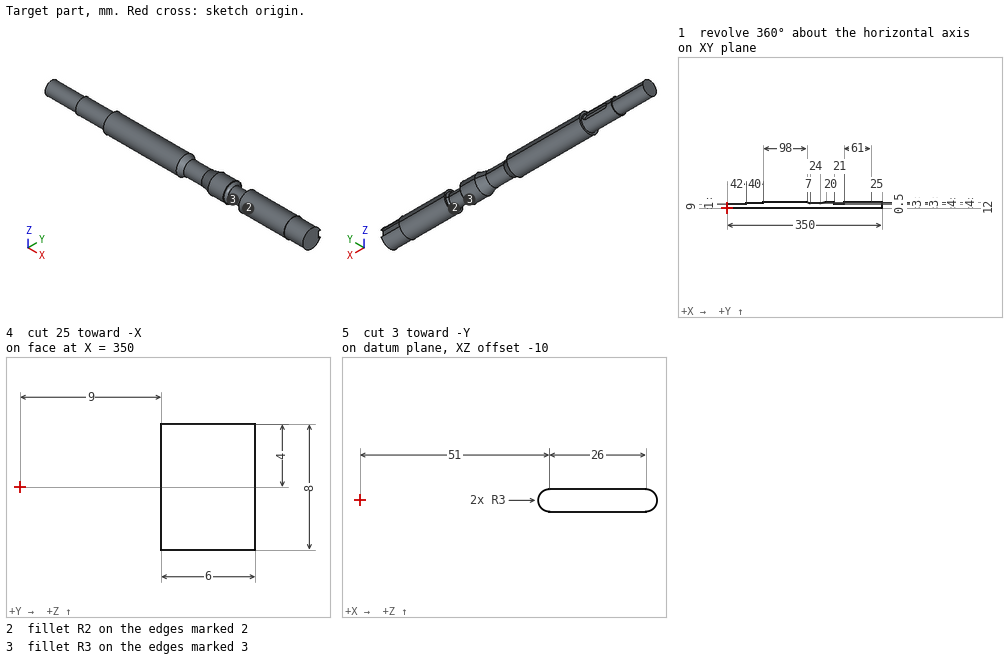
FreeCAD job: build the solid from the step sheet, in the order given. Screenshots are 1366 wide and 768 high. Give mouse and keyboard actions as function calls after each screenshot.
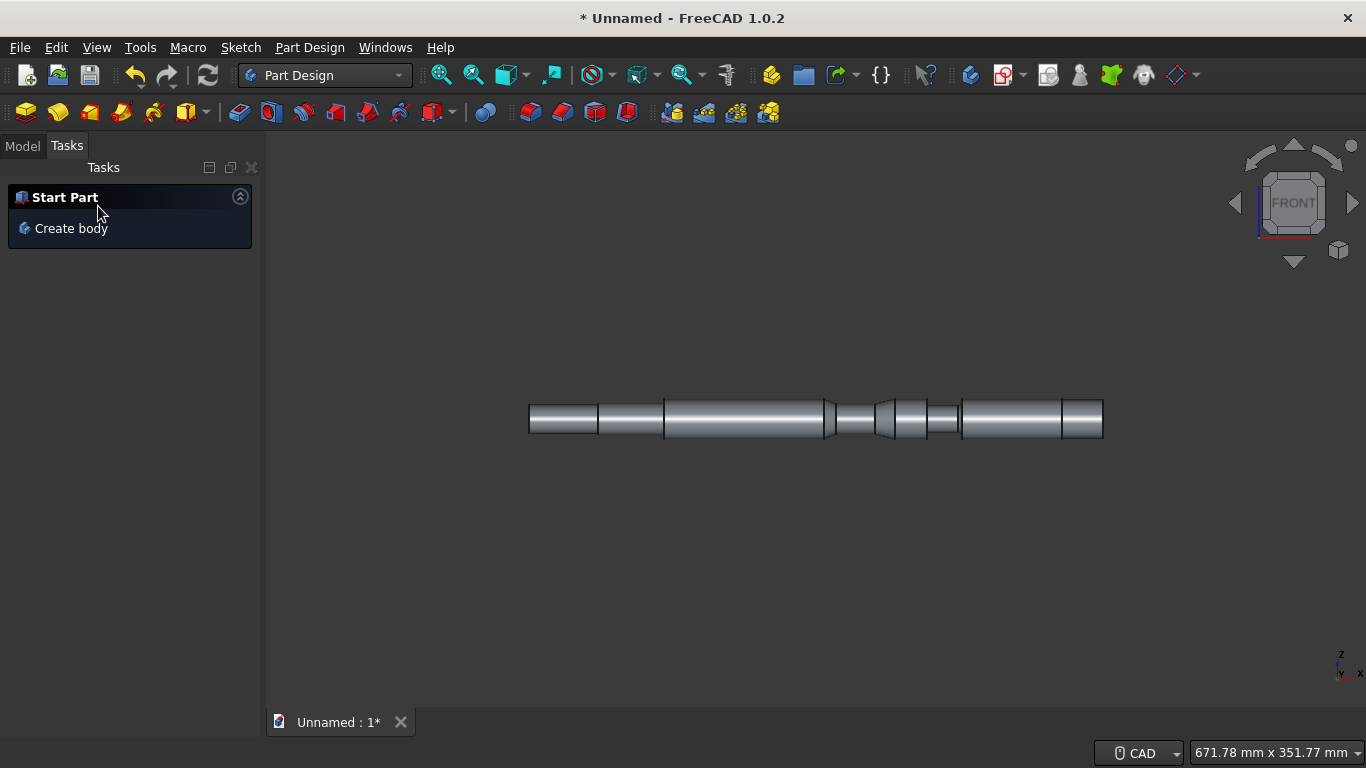
key(3)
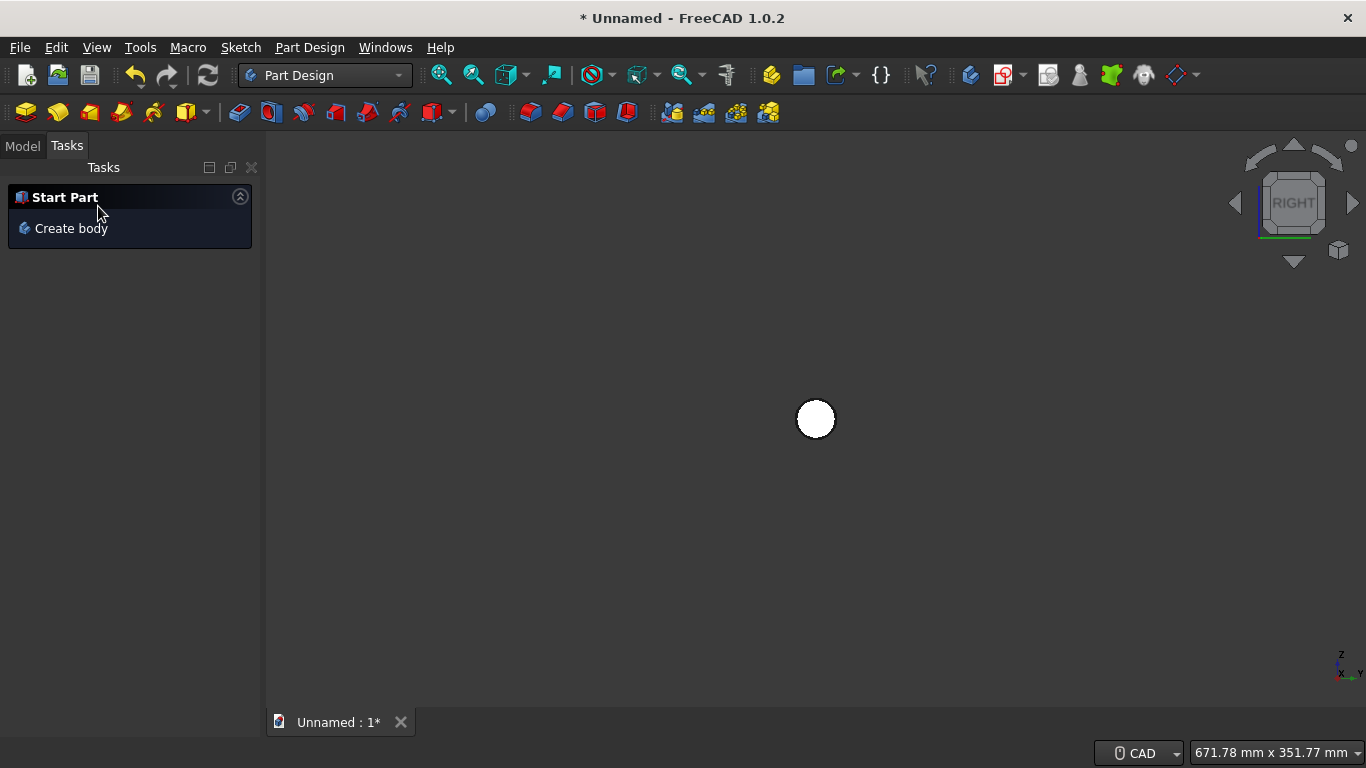
click(442, 76)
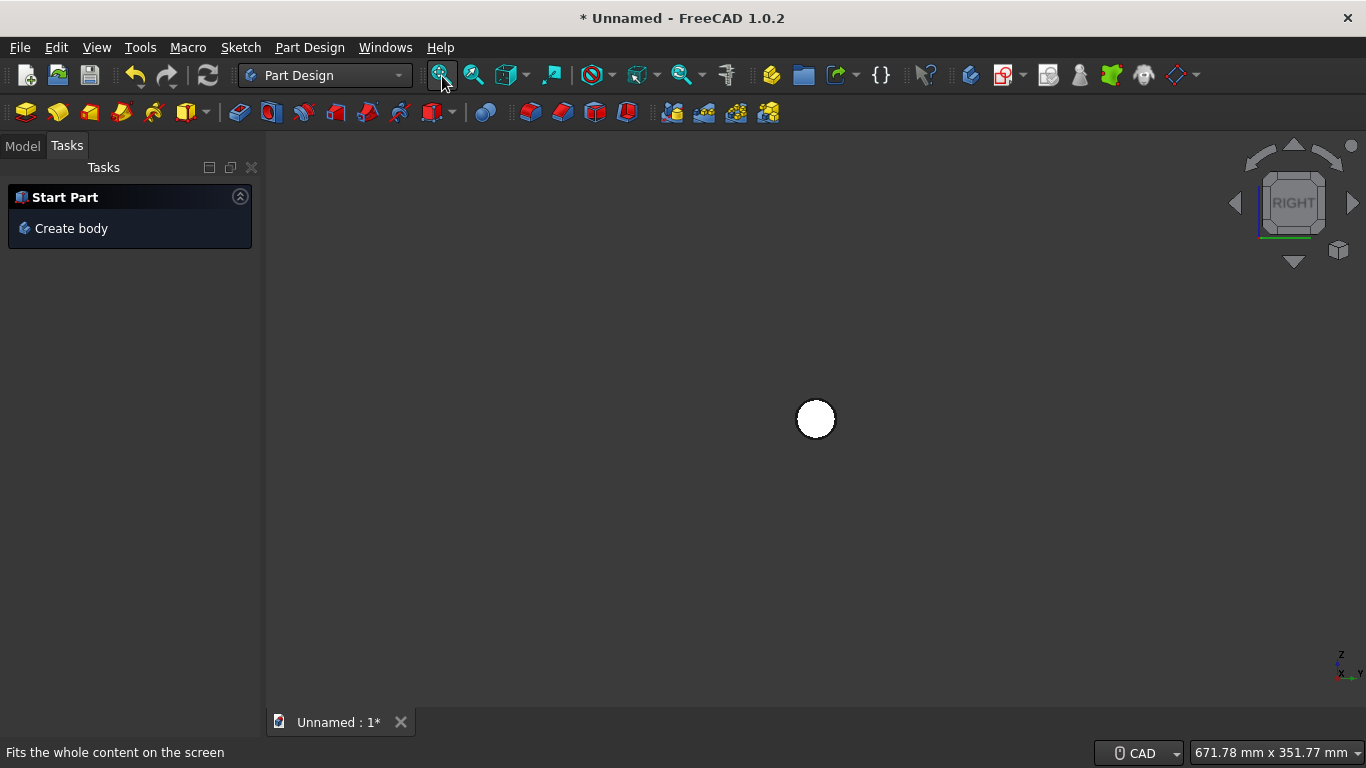
key(5)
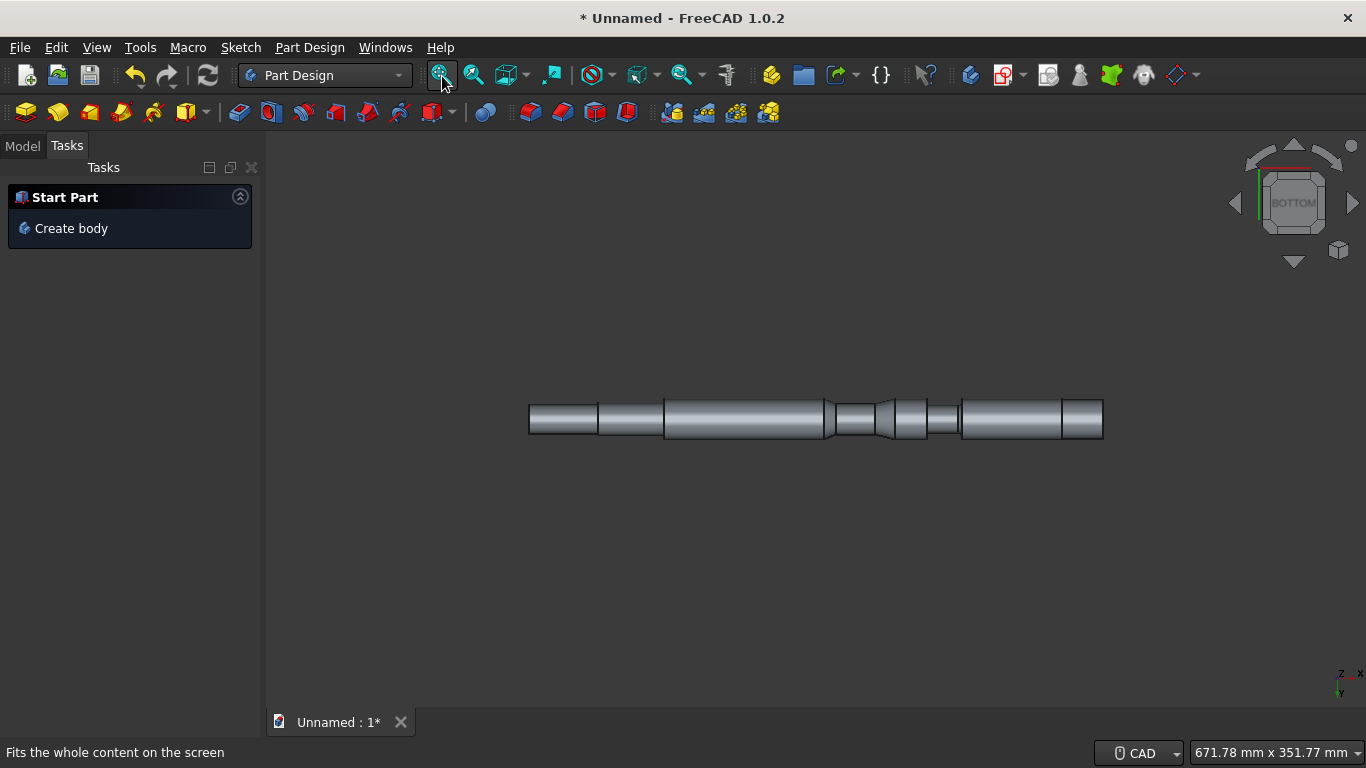
key(4)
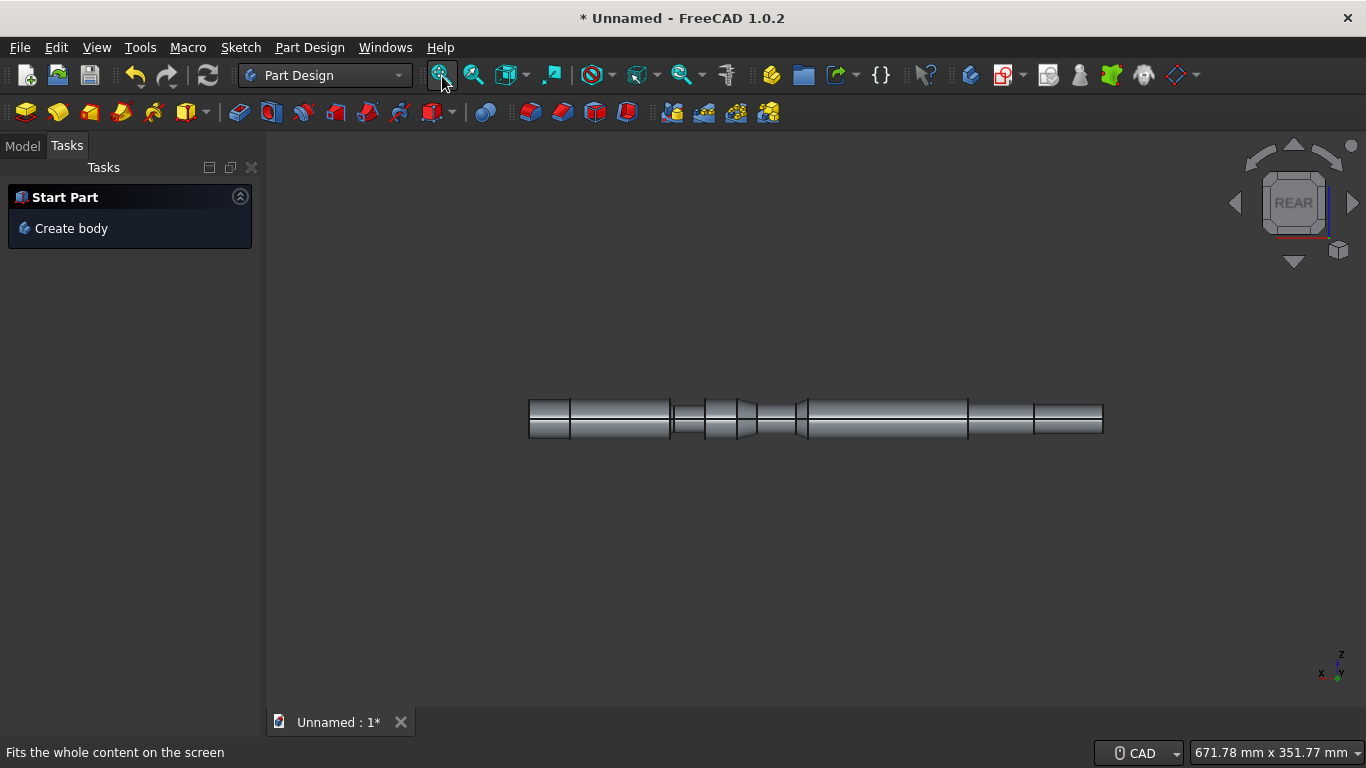
key(6)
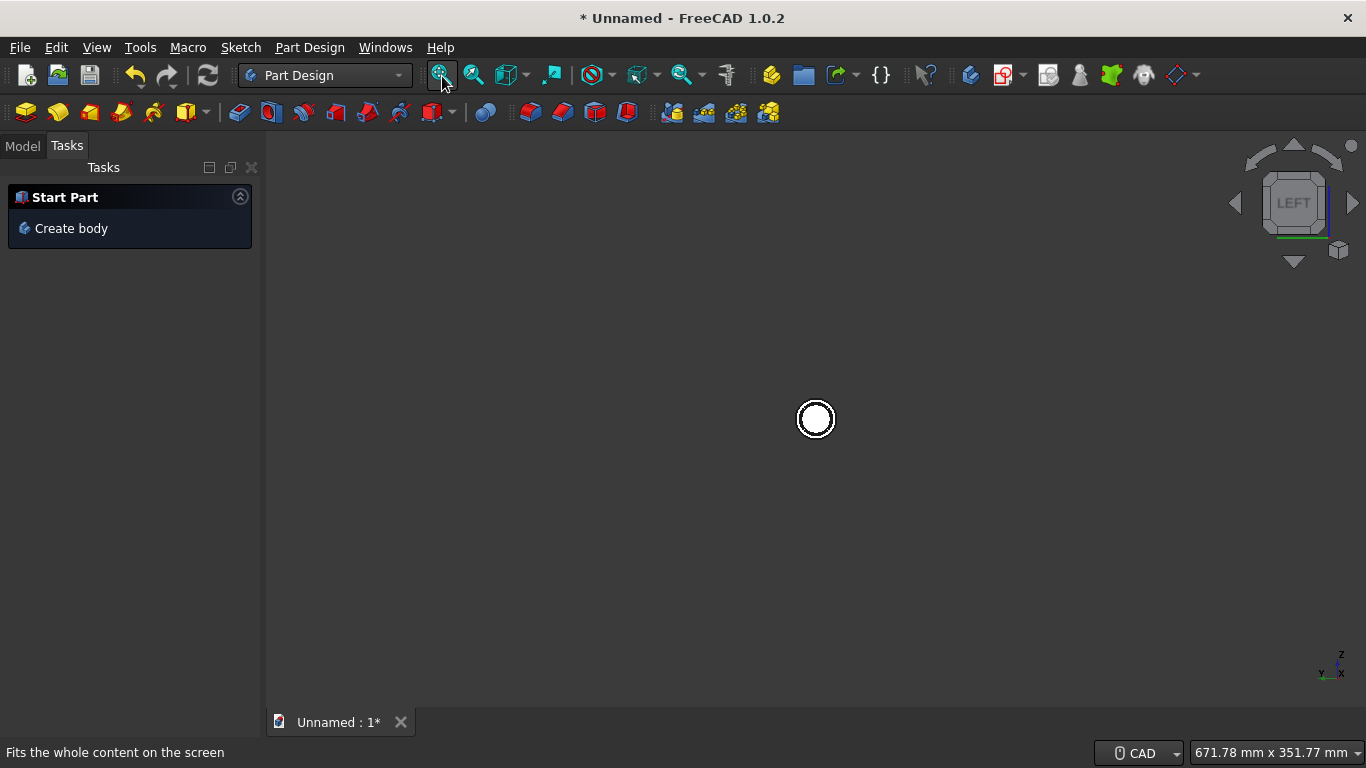
click(442, 76)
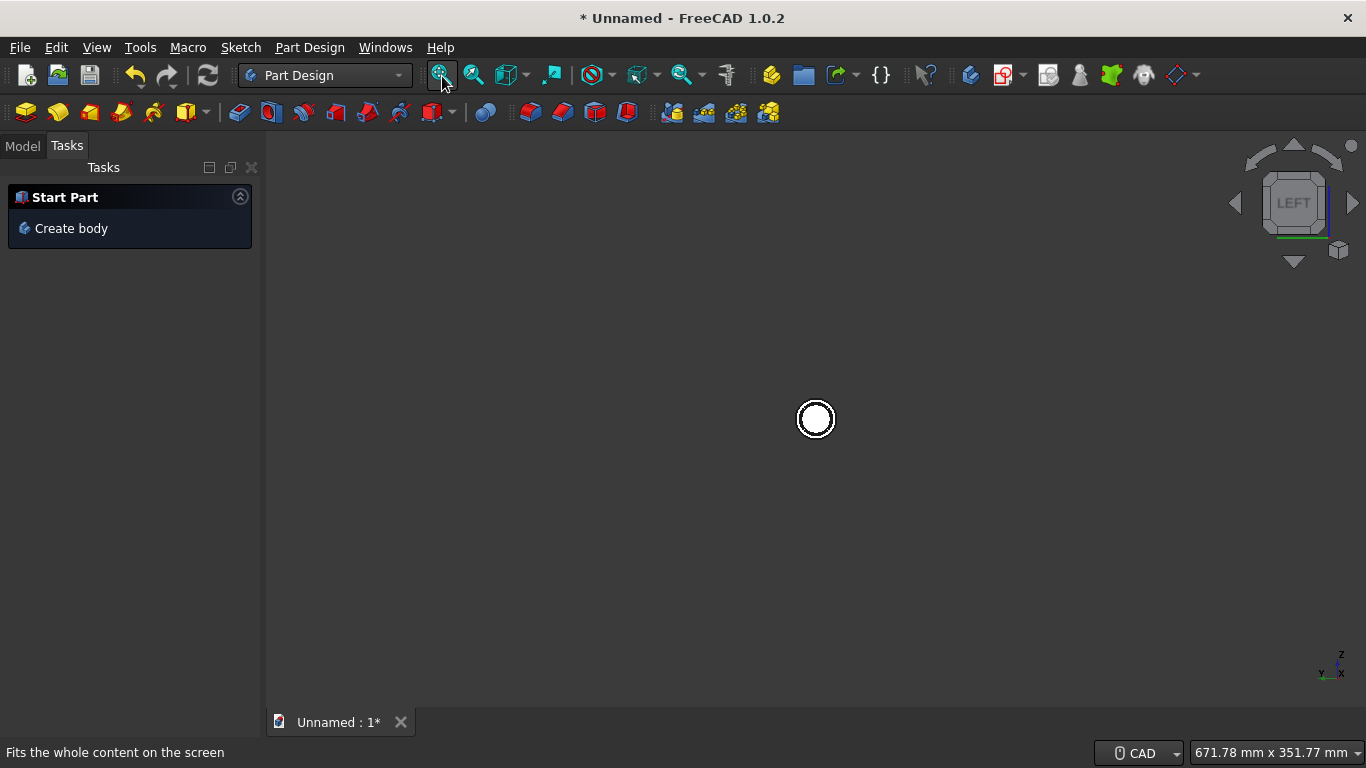
key(v)
key(3)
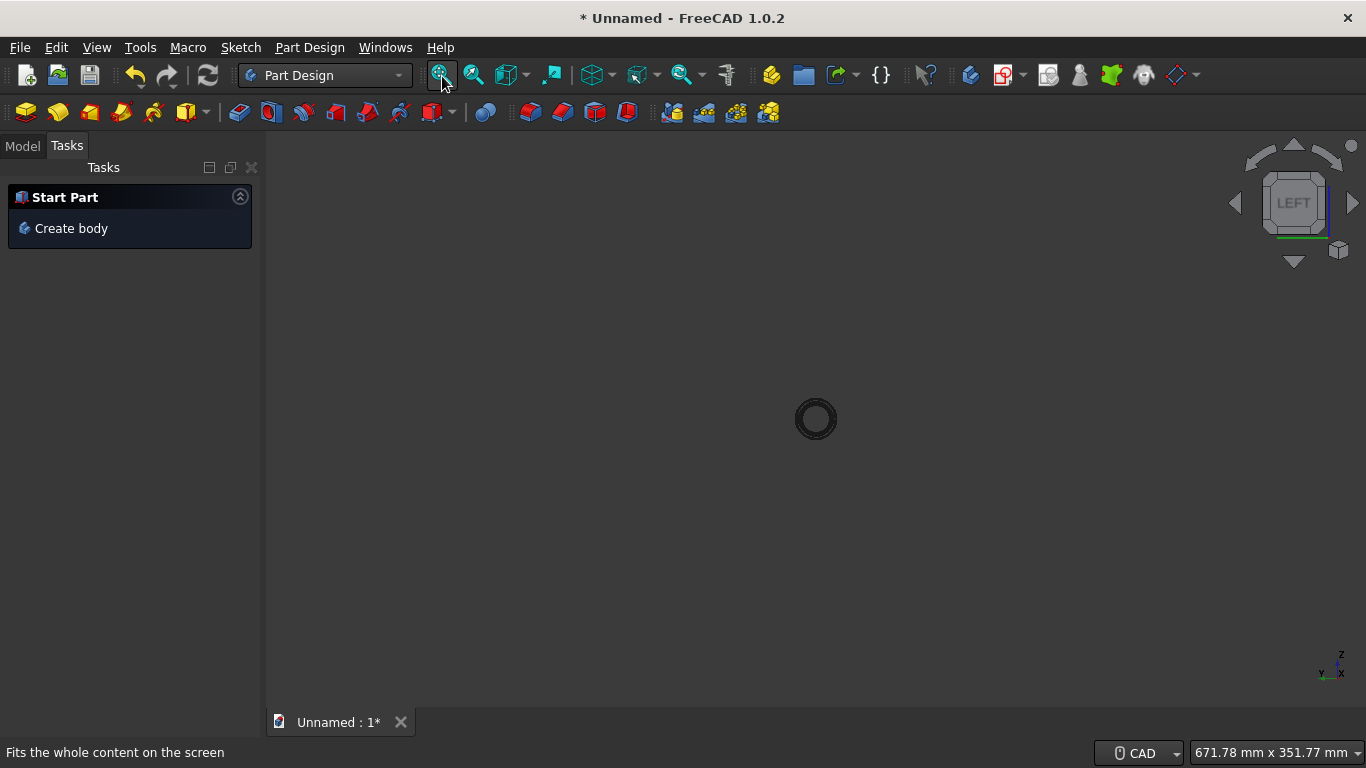
key(0)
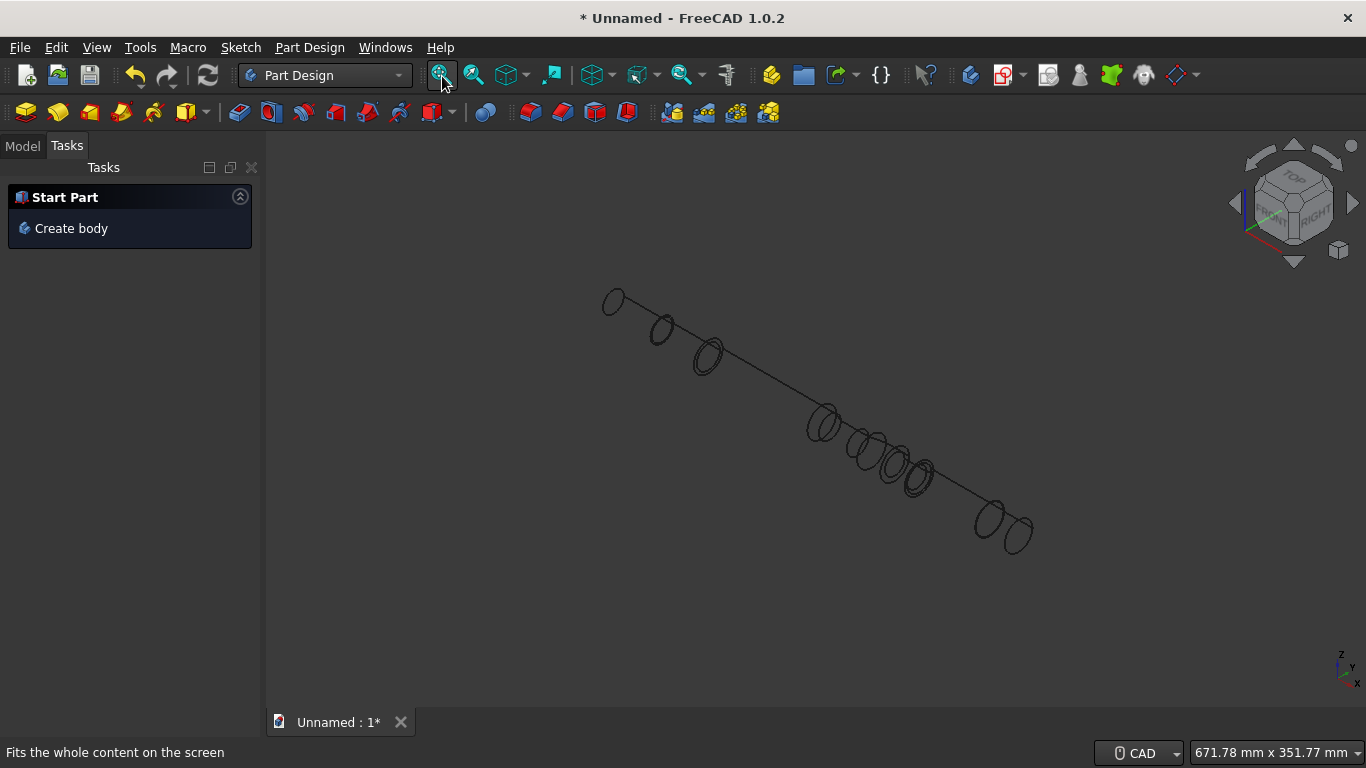
click(892, 476)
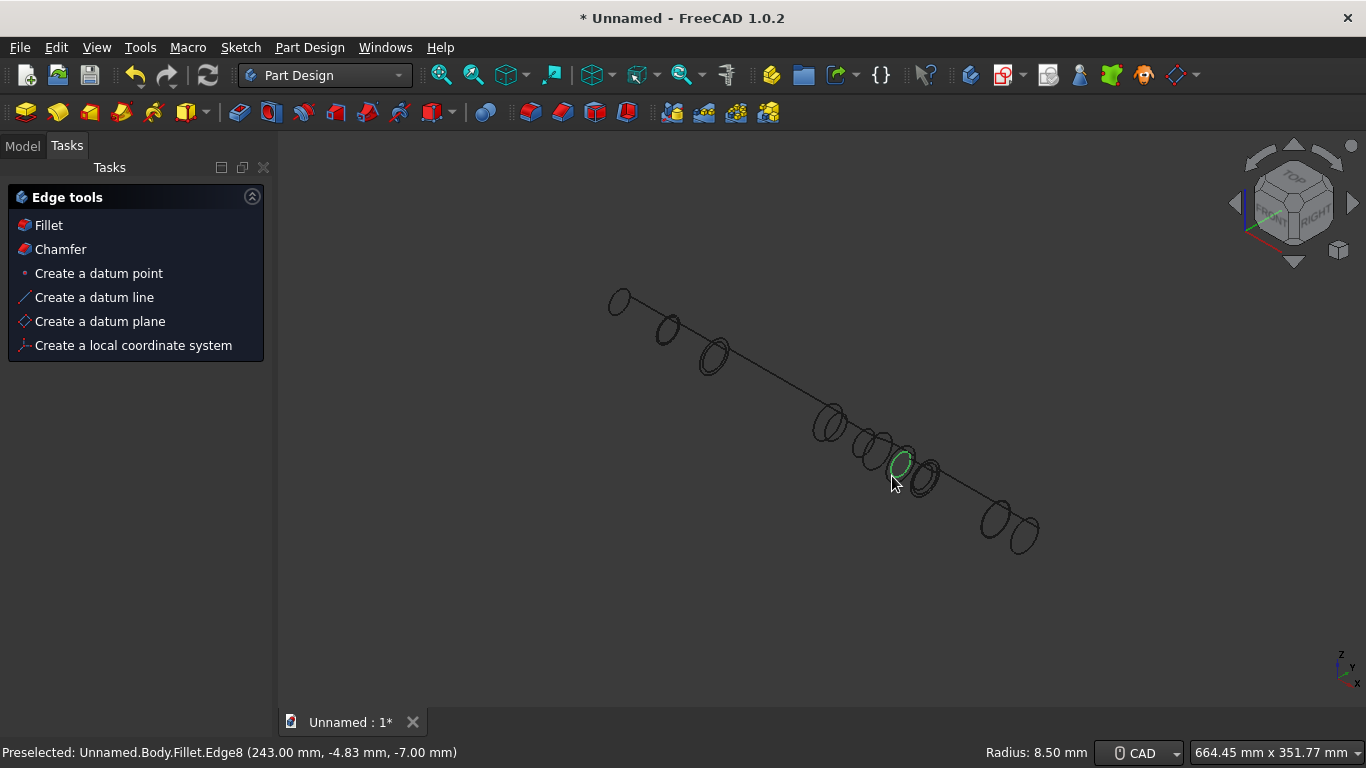
key(v)
key(1)